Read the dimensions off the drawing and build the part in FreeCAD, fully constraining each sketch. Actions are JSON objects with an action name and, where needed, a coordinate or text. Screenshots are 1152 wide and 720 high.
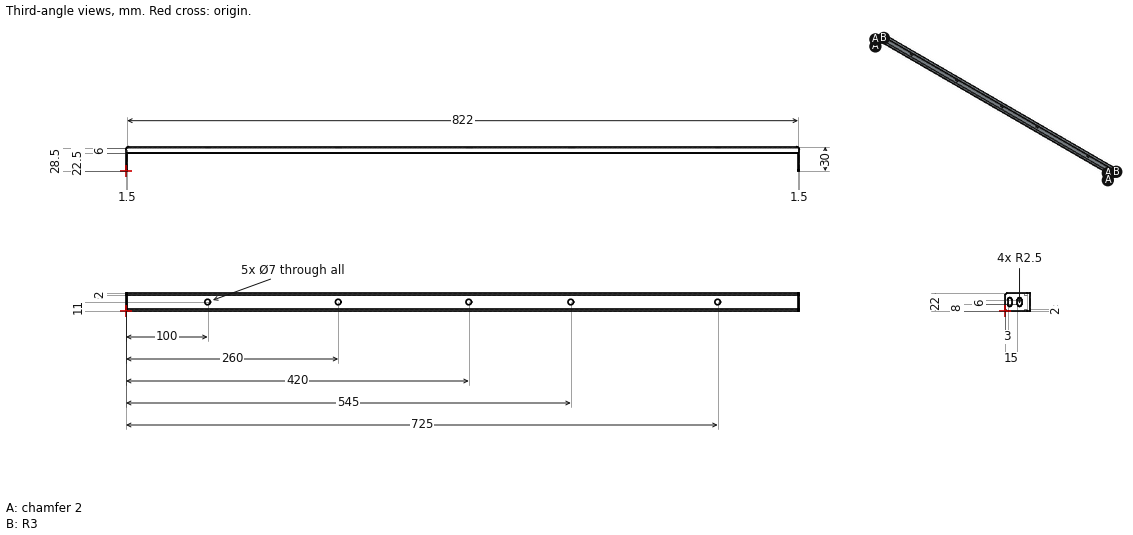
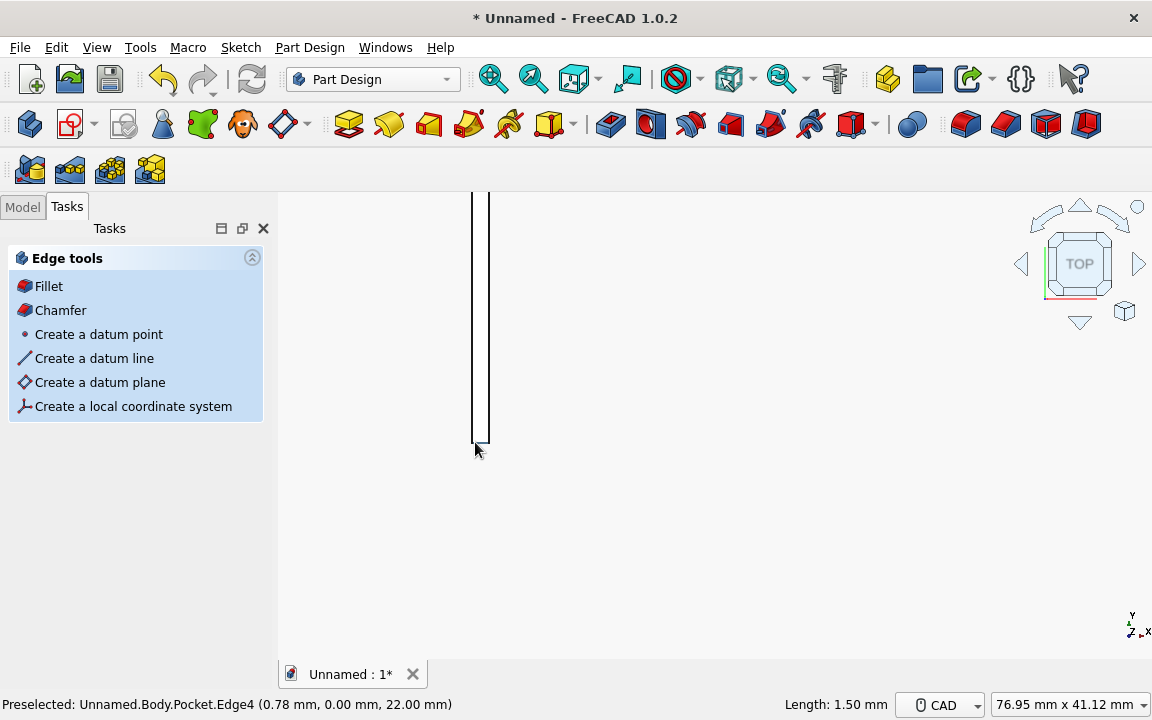
{"action": "scroll", "coordinate": [481, 442], "scroll_direction": "up", "scroll_amount": 5}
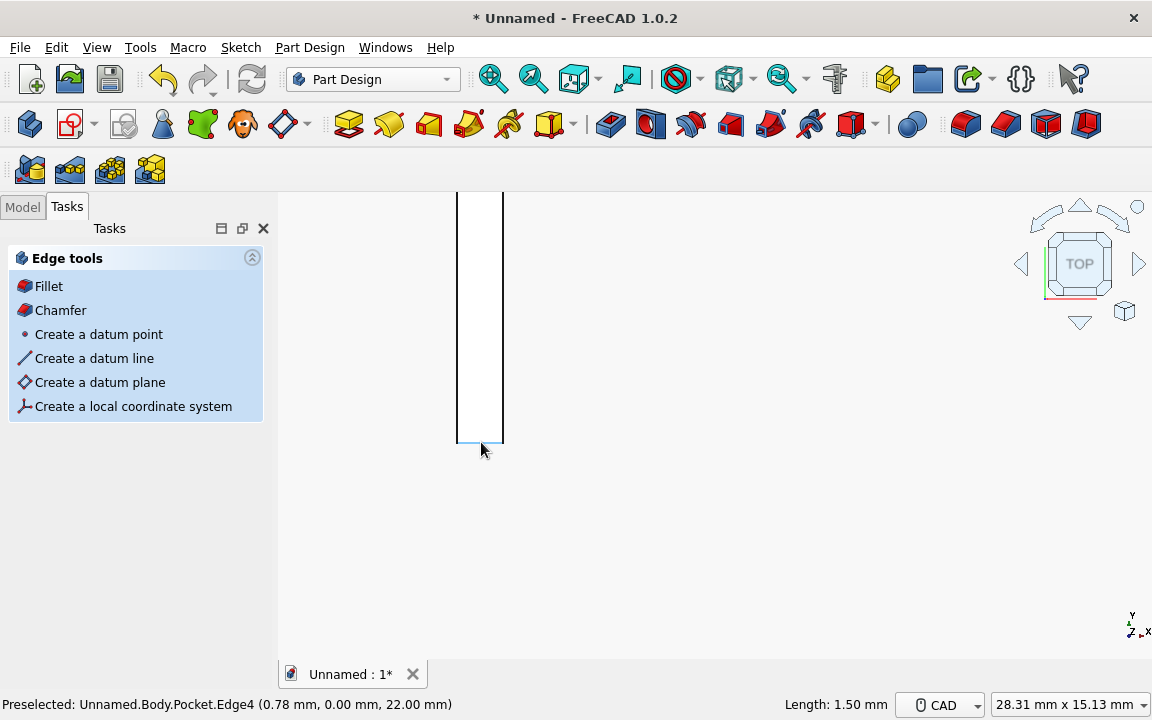
{"action": "left_click", "coordinate": [494, 80]}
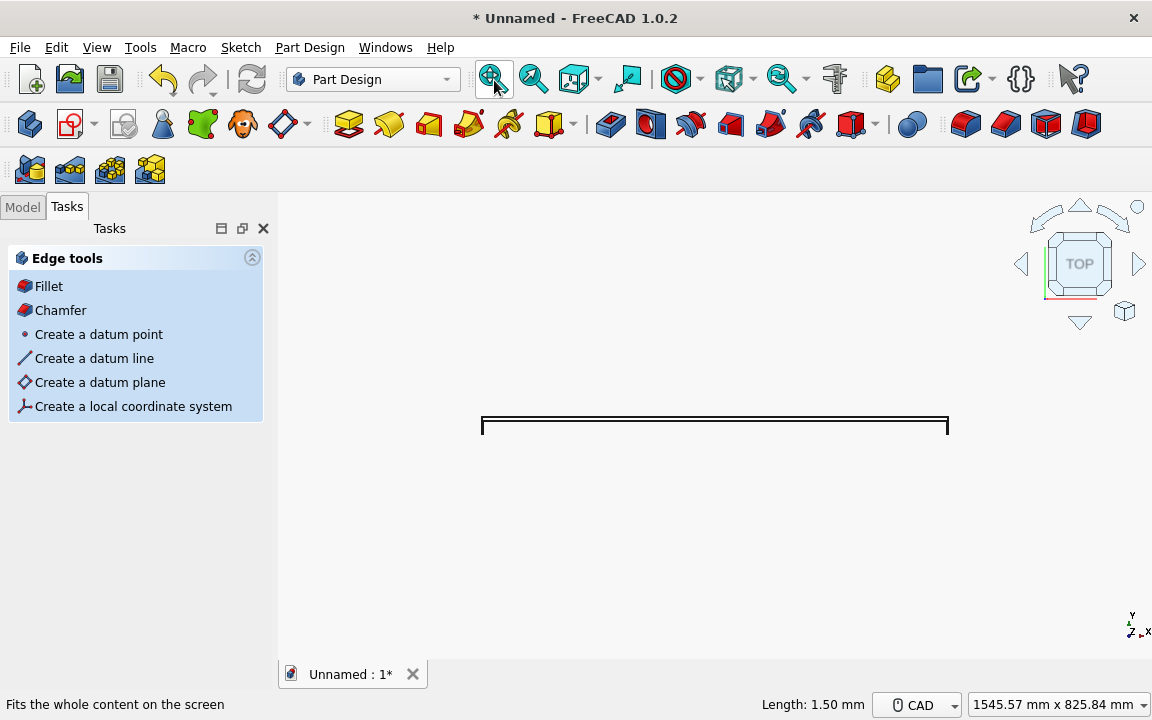
{"action": "key", "text": "1"}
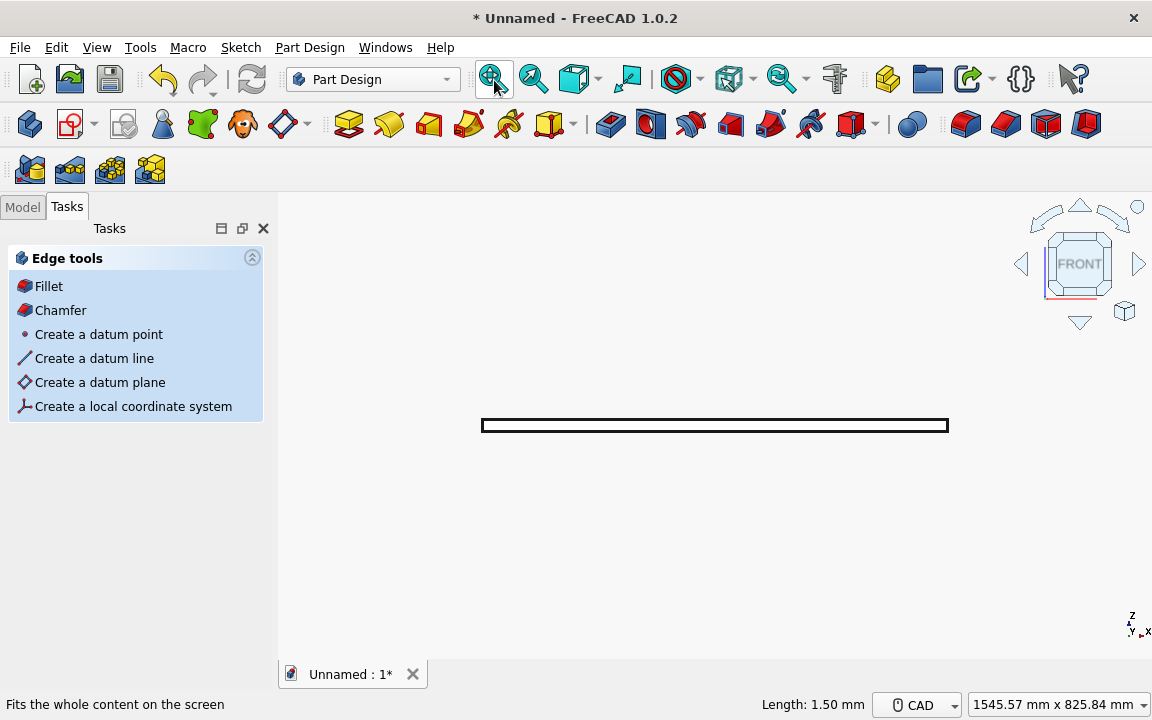
{"action": "scroll", "coordinate": [482, 431], "scroll_direction": "up", "scroll_amount": 15}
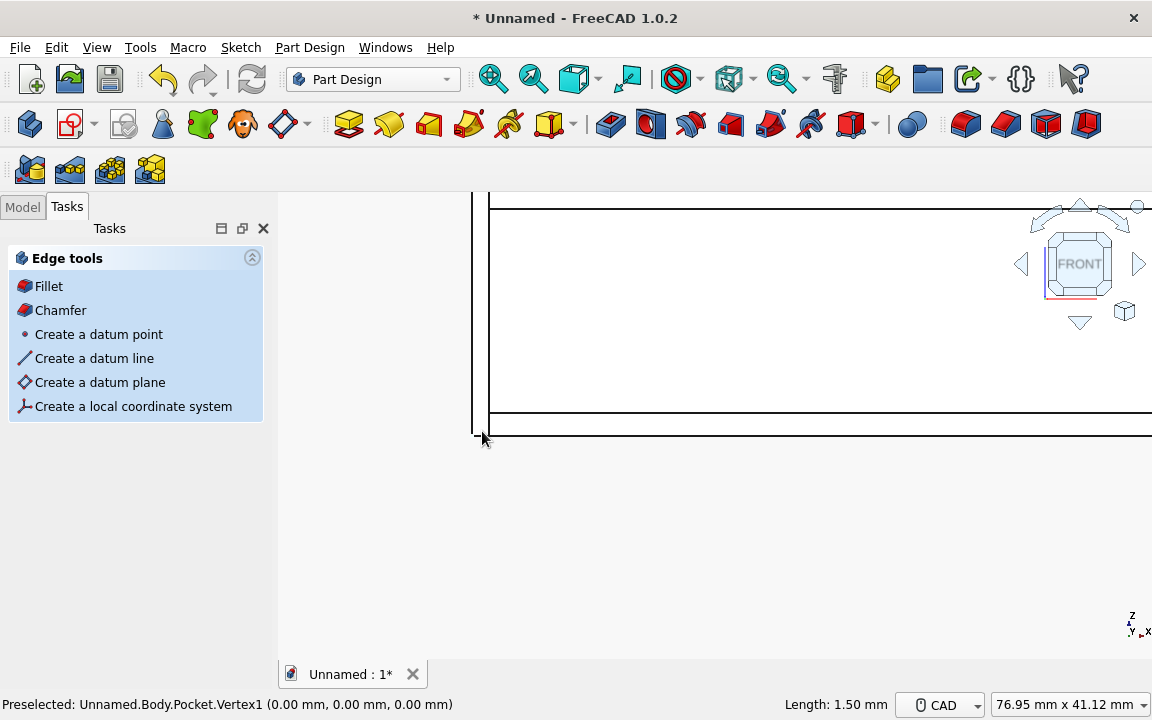
{"action": "left_click", "coordinate": [481, 435], "text": "ctrl"}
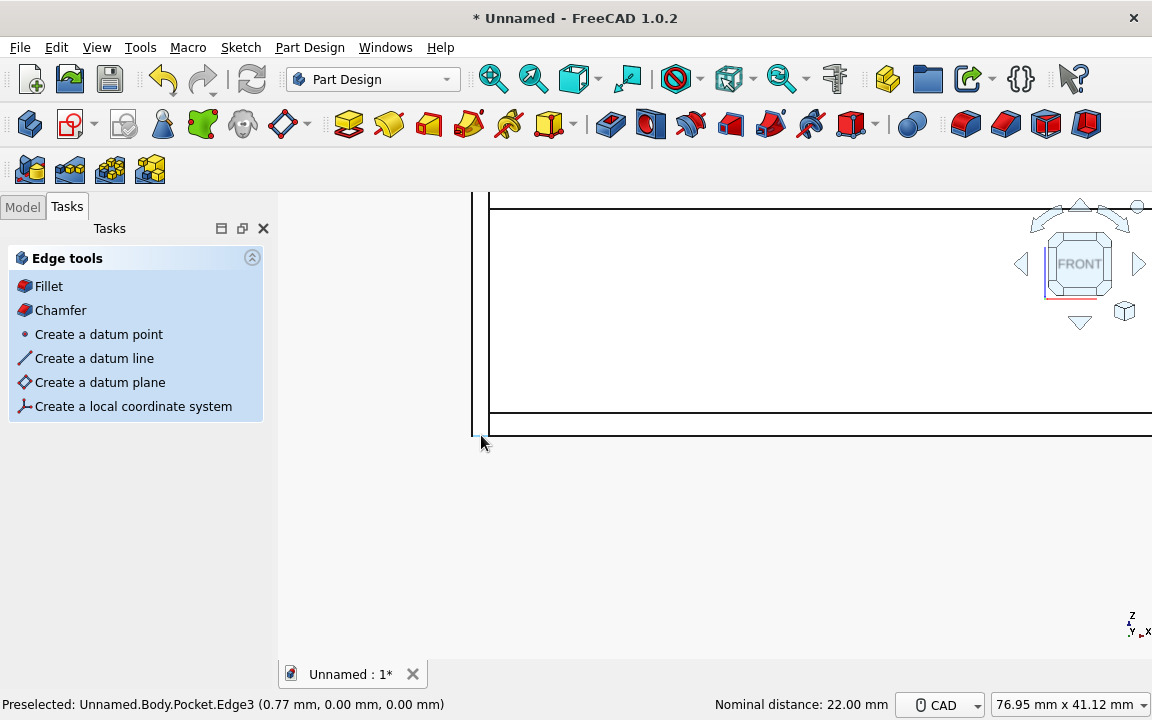
{"action": "left_click", "coordinate": [494, 80]}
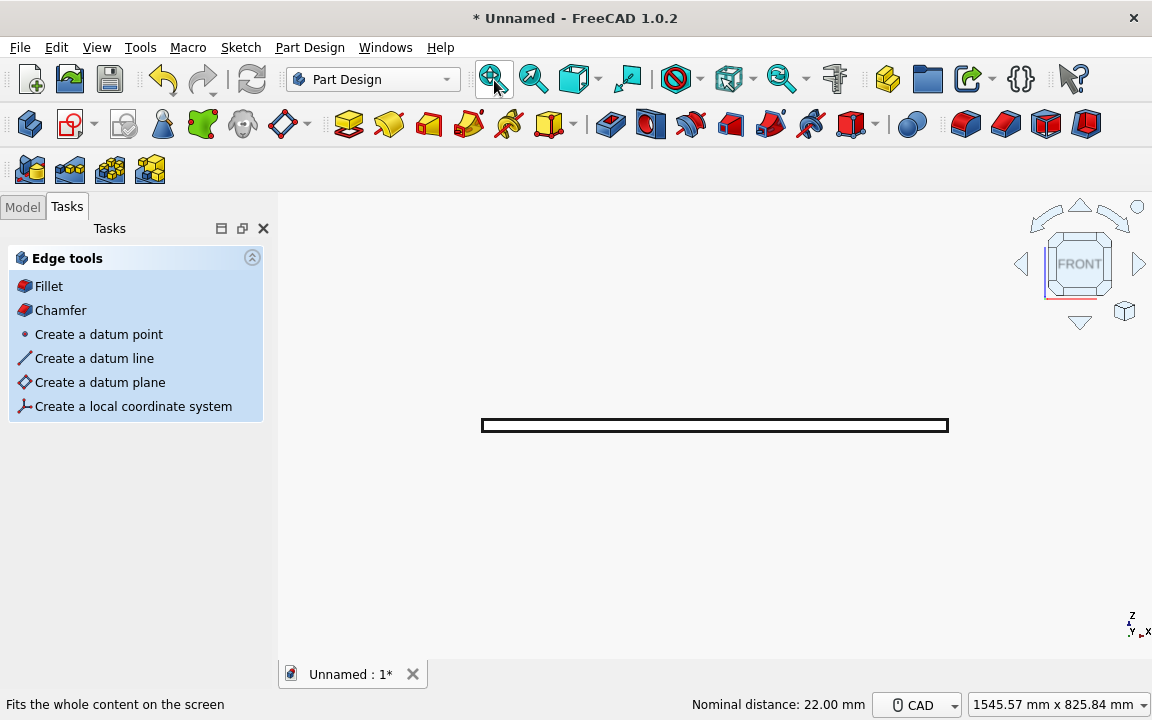
{"action": "key", "text": "3"}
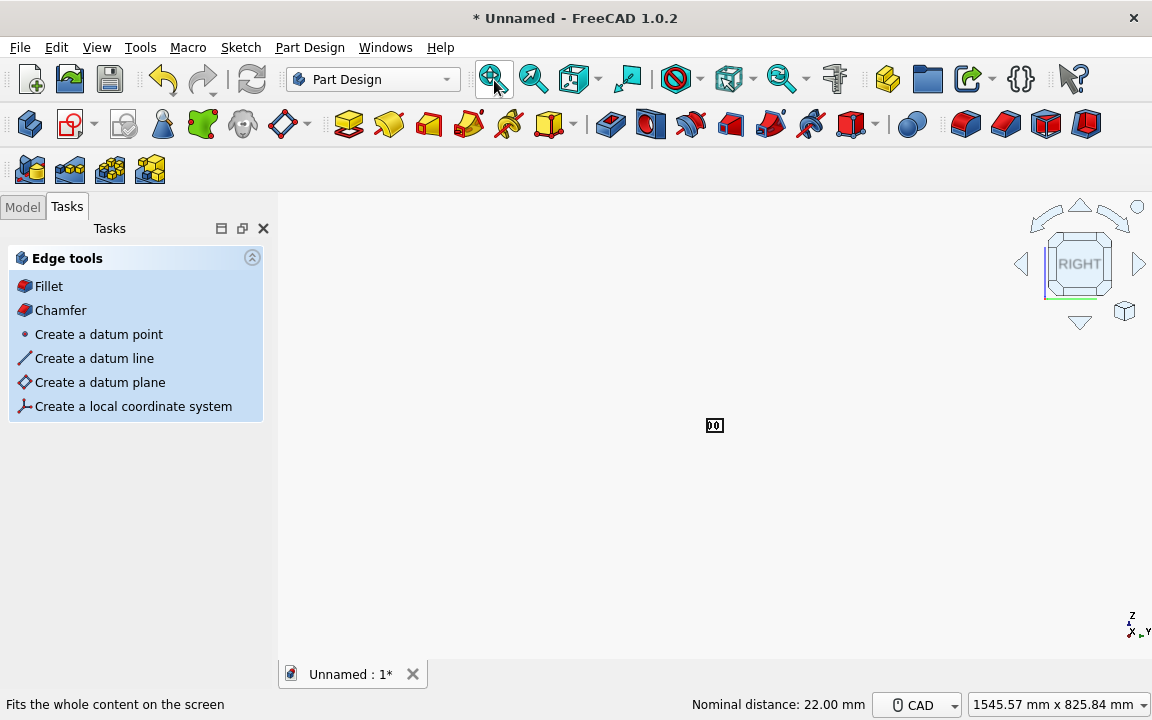
{"action": "left_click", "coordinate": [494, 80]}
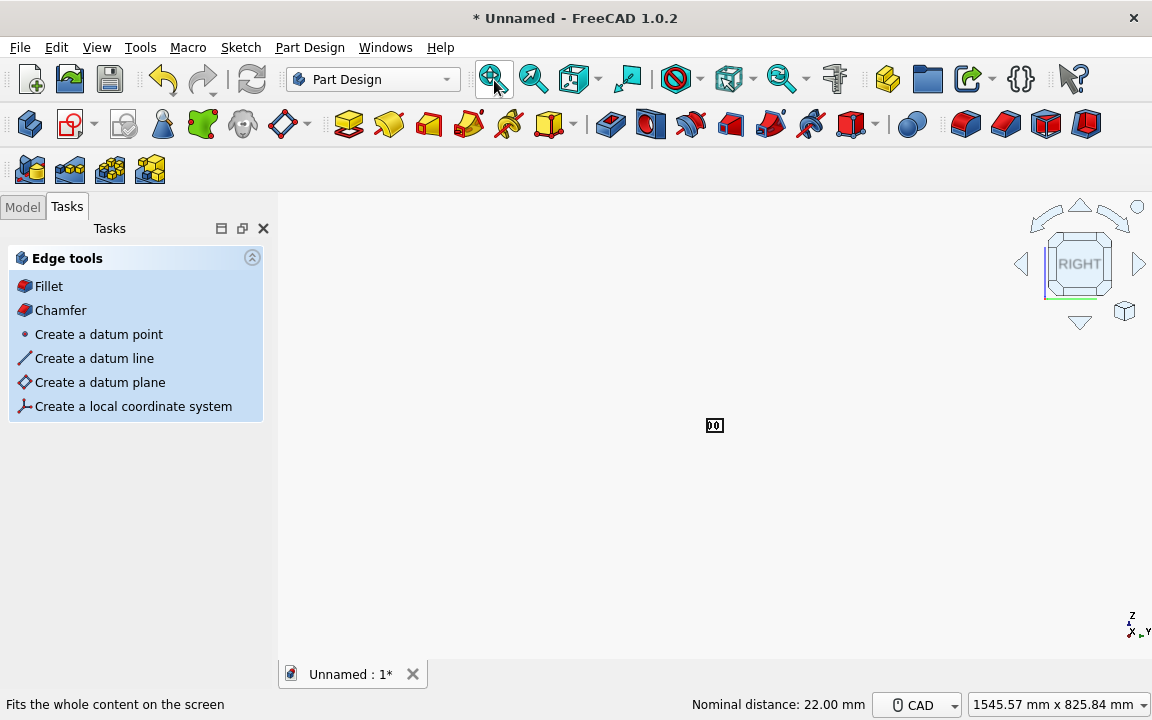
{"action": "scroll", "coordinate": [707, 418], "scroll_direction": "up", "scroll_amount": 15}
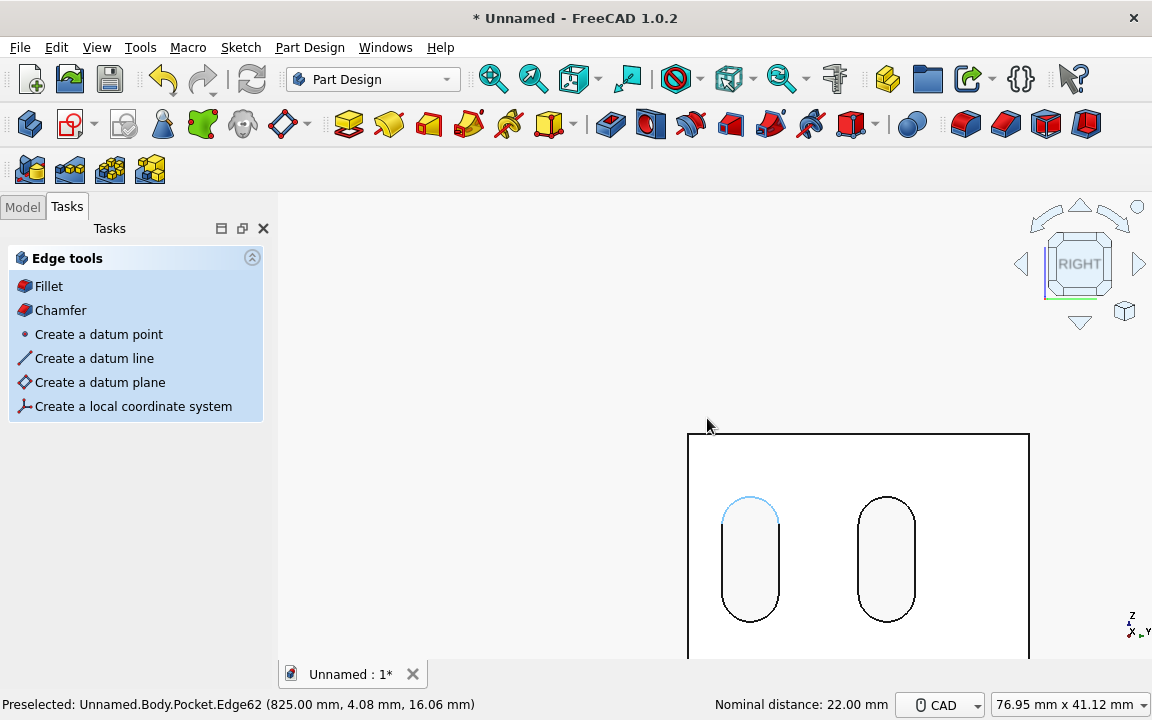
{"action": "scroll", "coordinate": [688, 433], "scroll_direction": "up", "scroll_amount": 5}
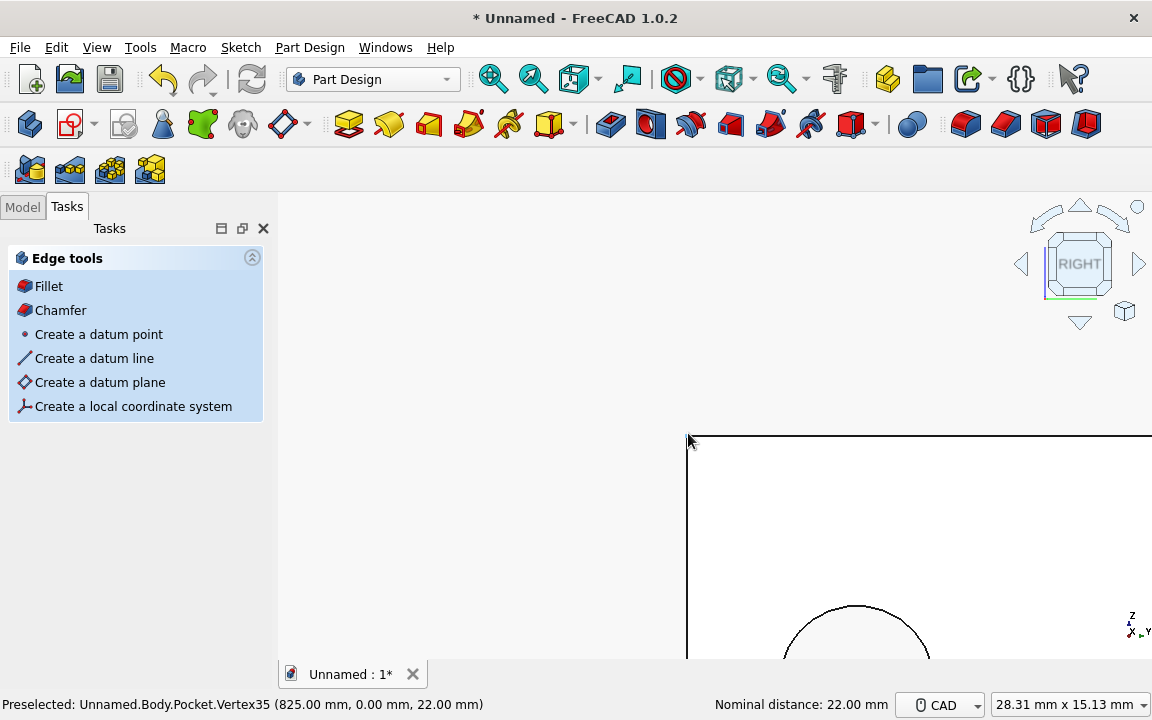
{"action": "left_click", "coordinate": [494, 80]}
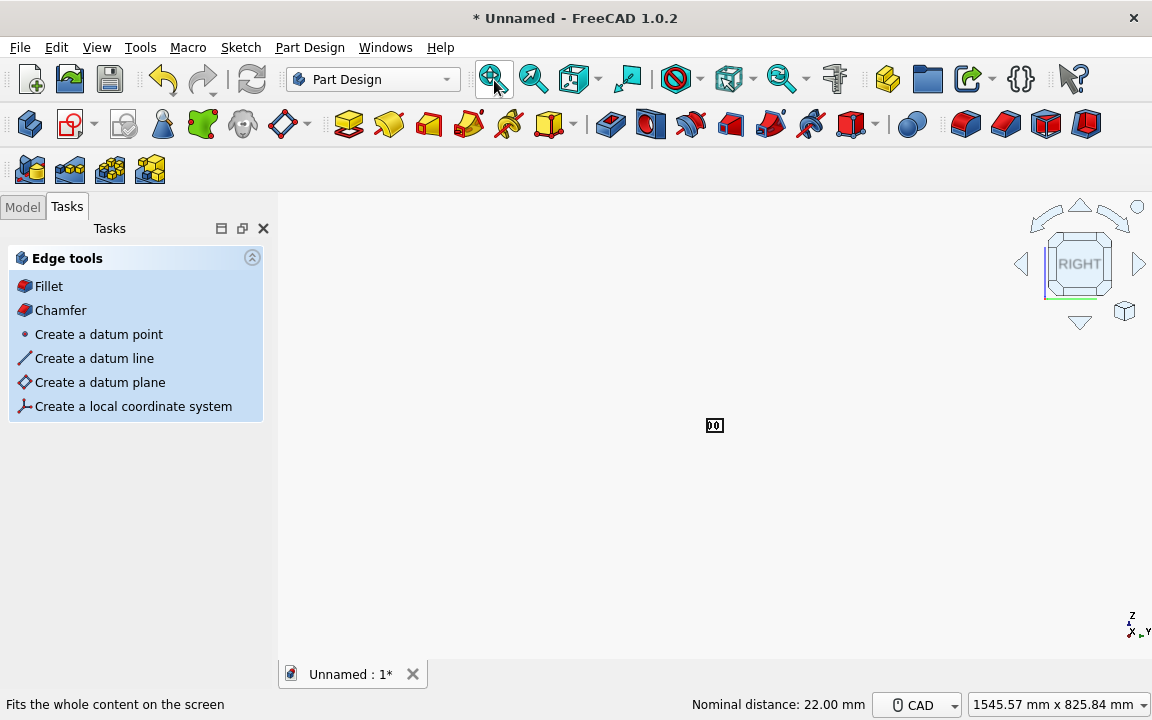
{"action": "key", "text": "5"}